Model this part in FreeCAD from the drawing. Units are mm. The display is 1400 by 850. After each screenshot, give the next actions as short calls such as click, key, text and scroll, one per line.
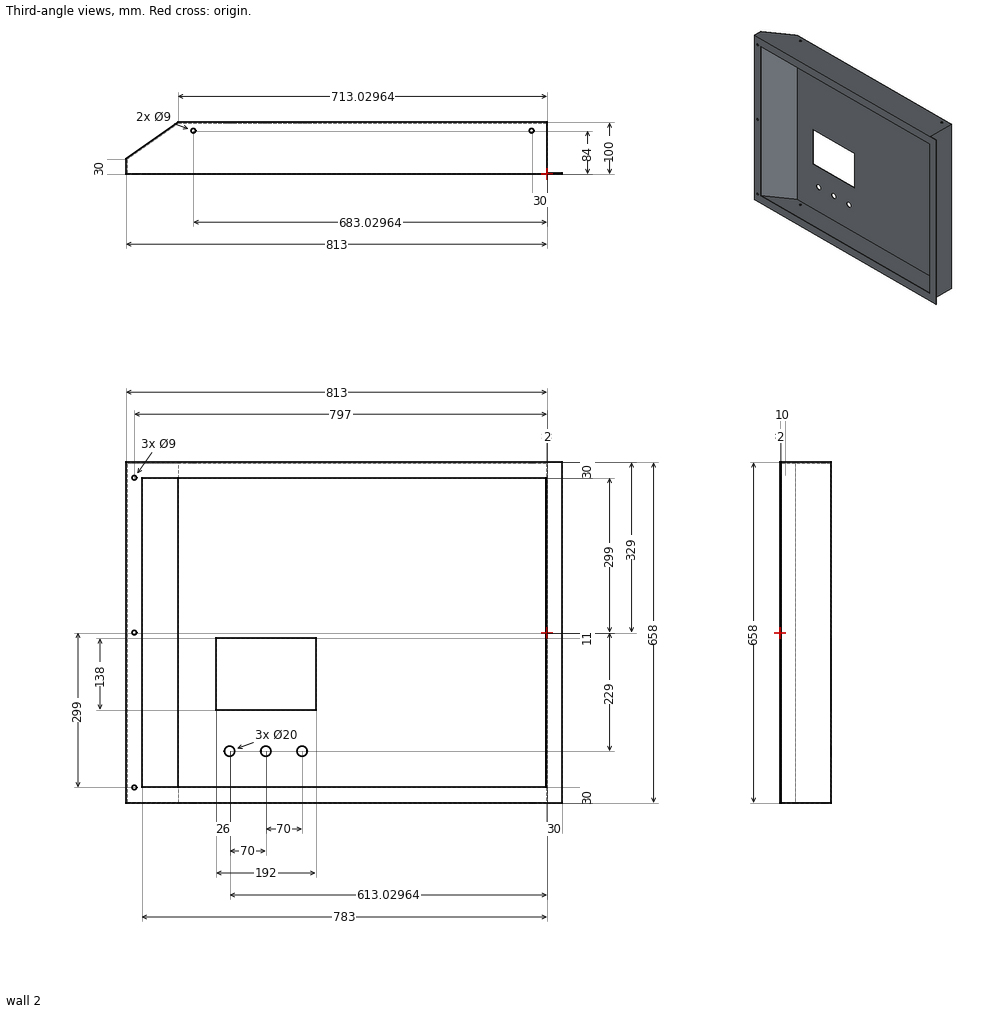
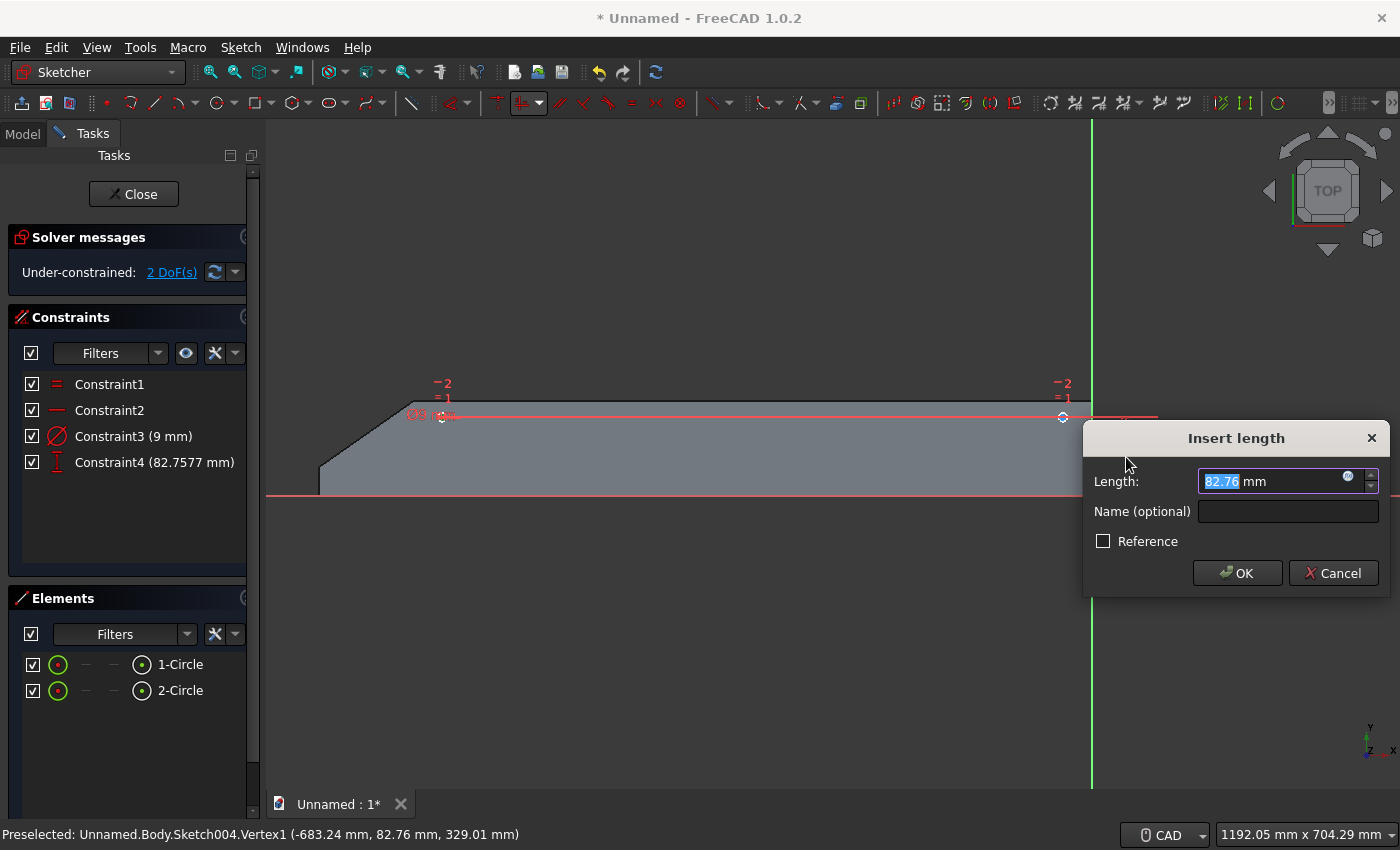
text(84)
key(Return)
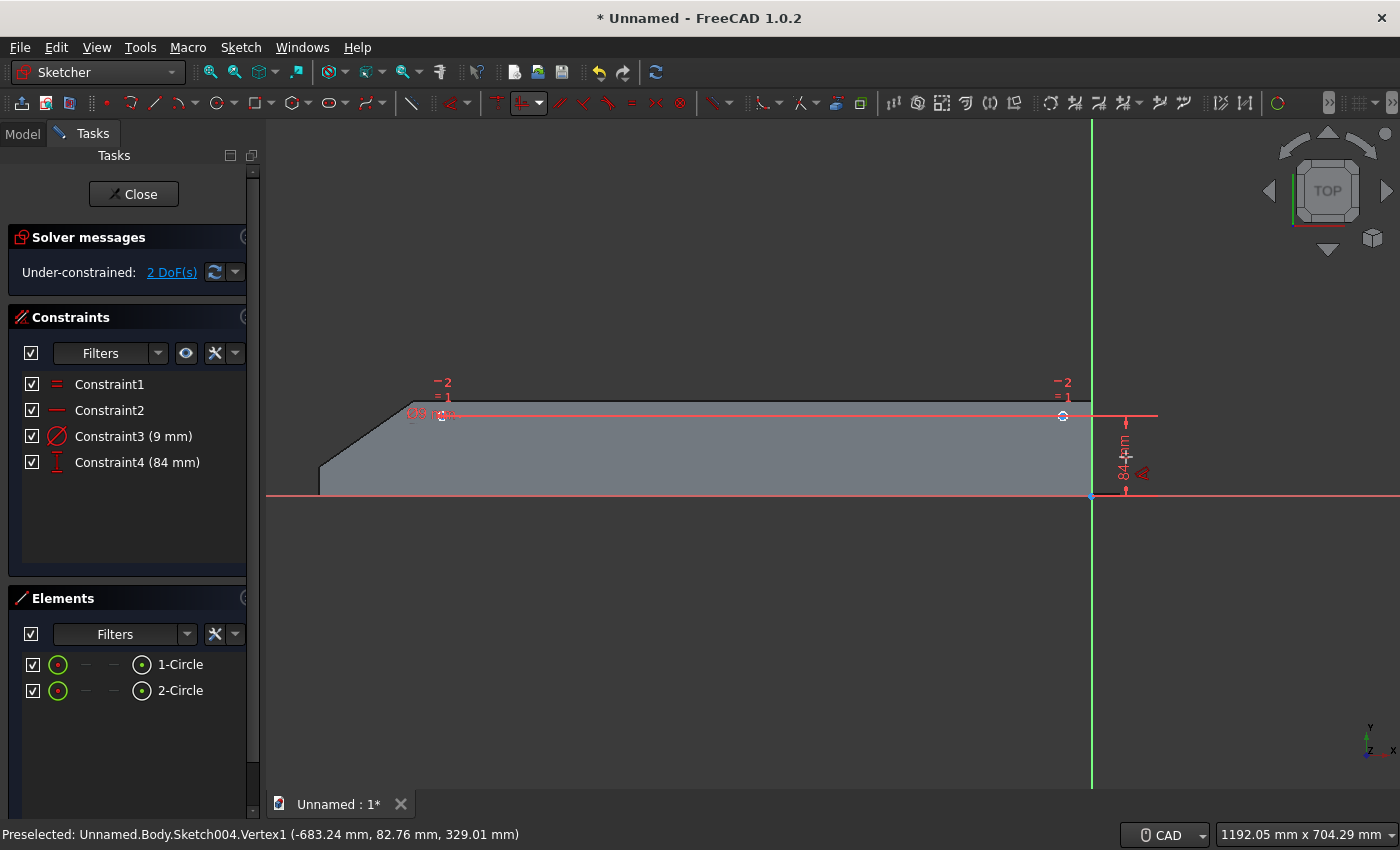
scroll(1063, 416, up, 2)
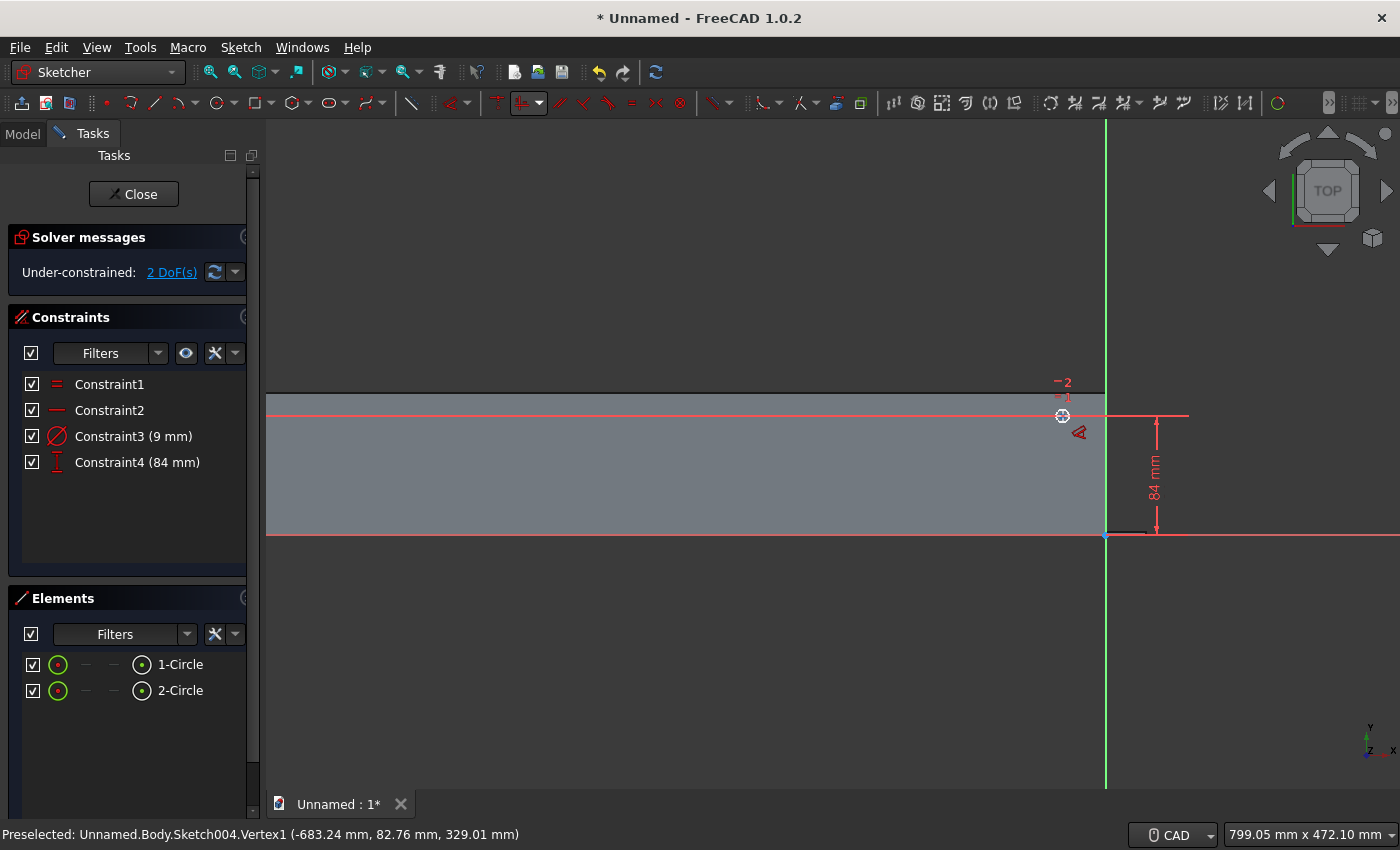
click(1063, 416)
click(1084, 569)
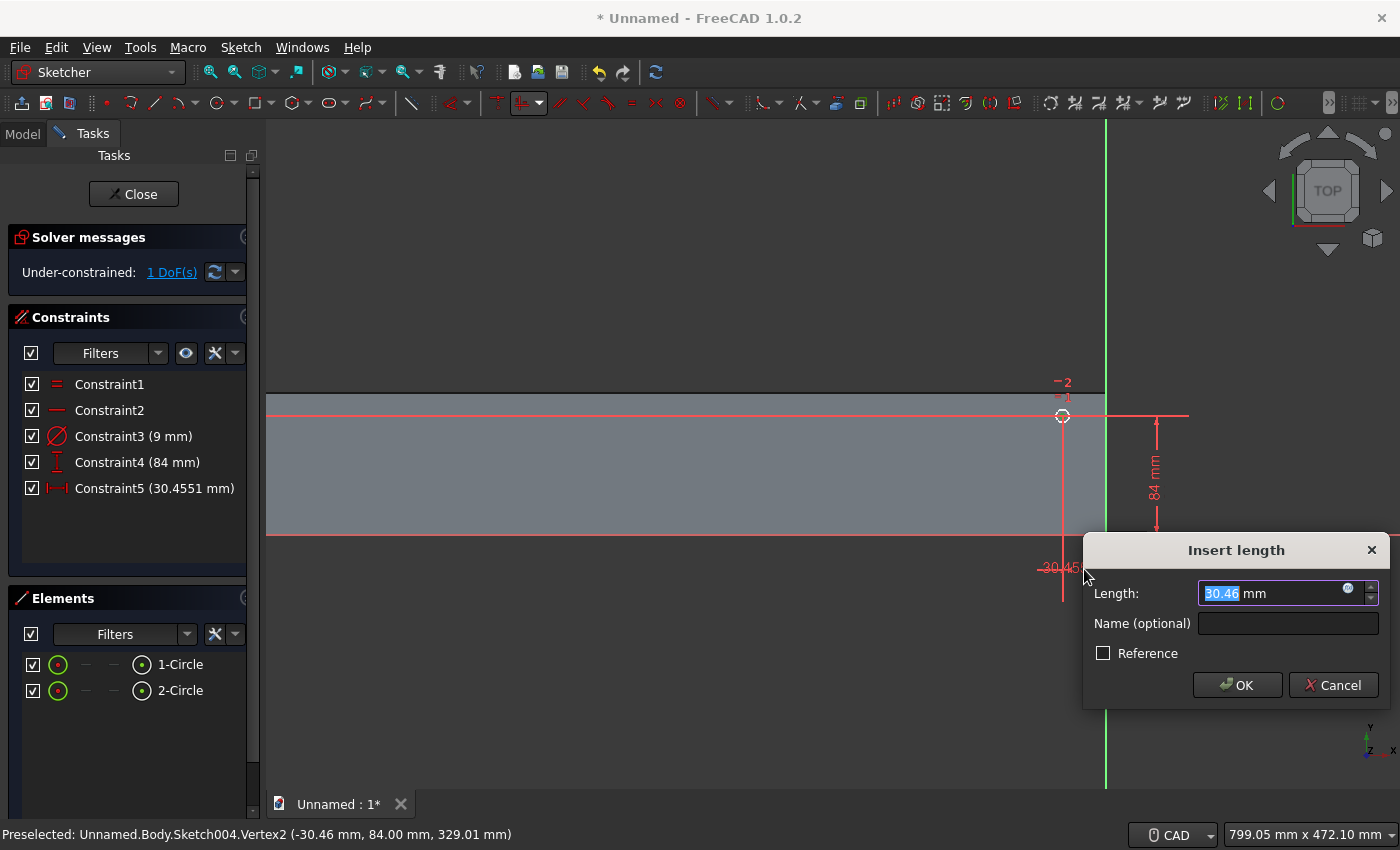
text(30)
key(Return)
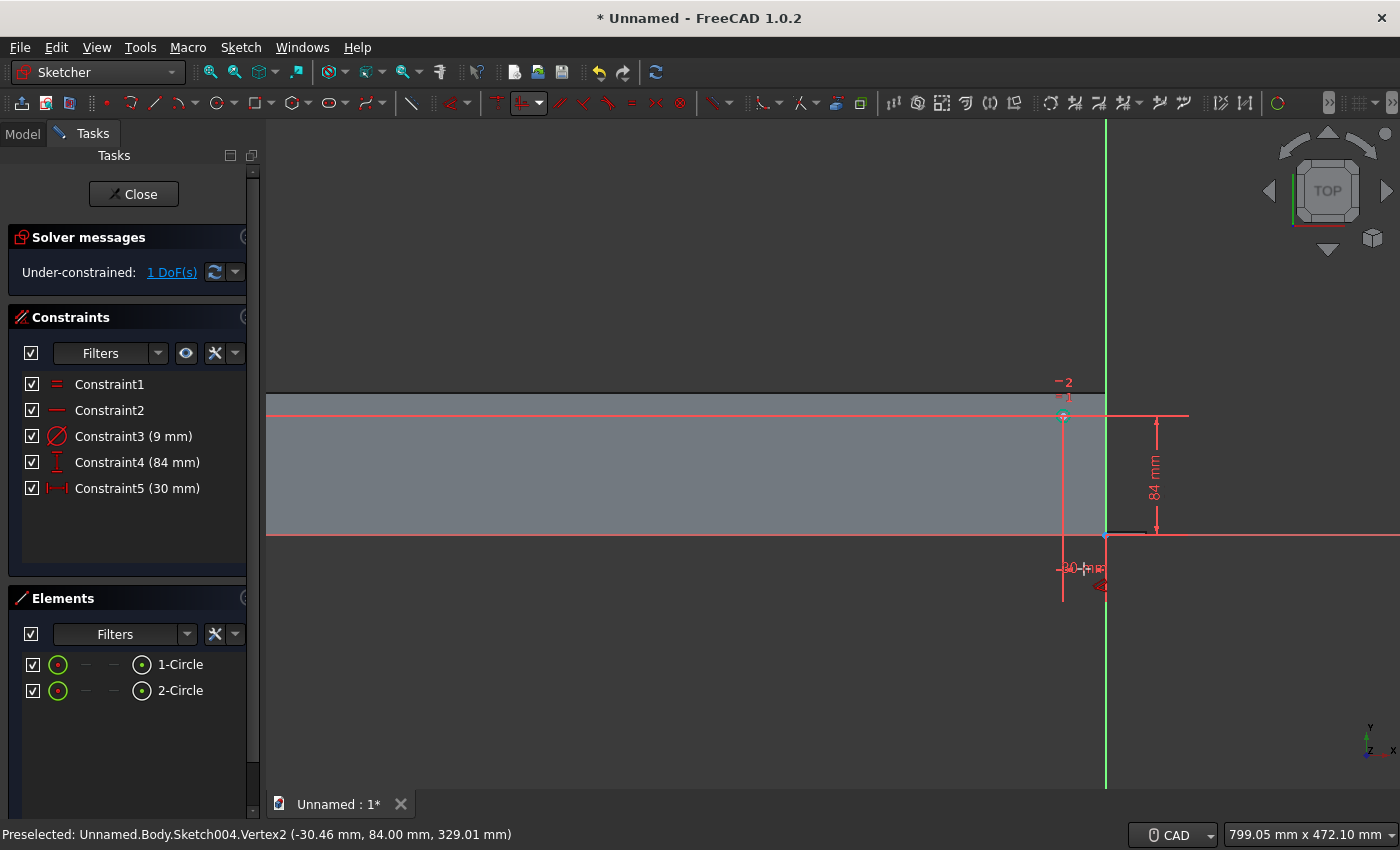
scroll(1062, 416, down, 2)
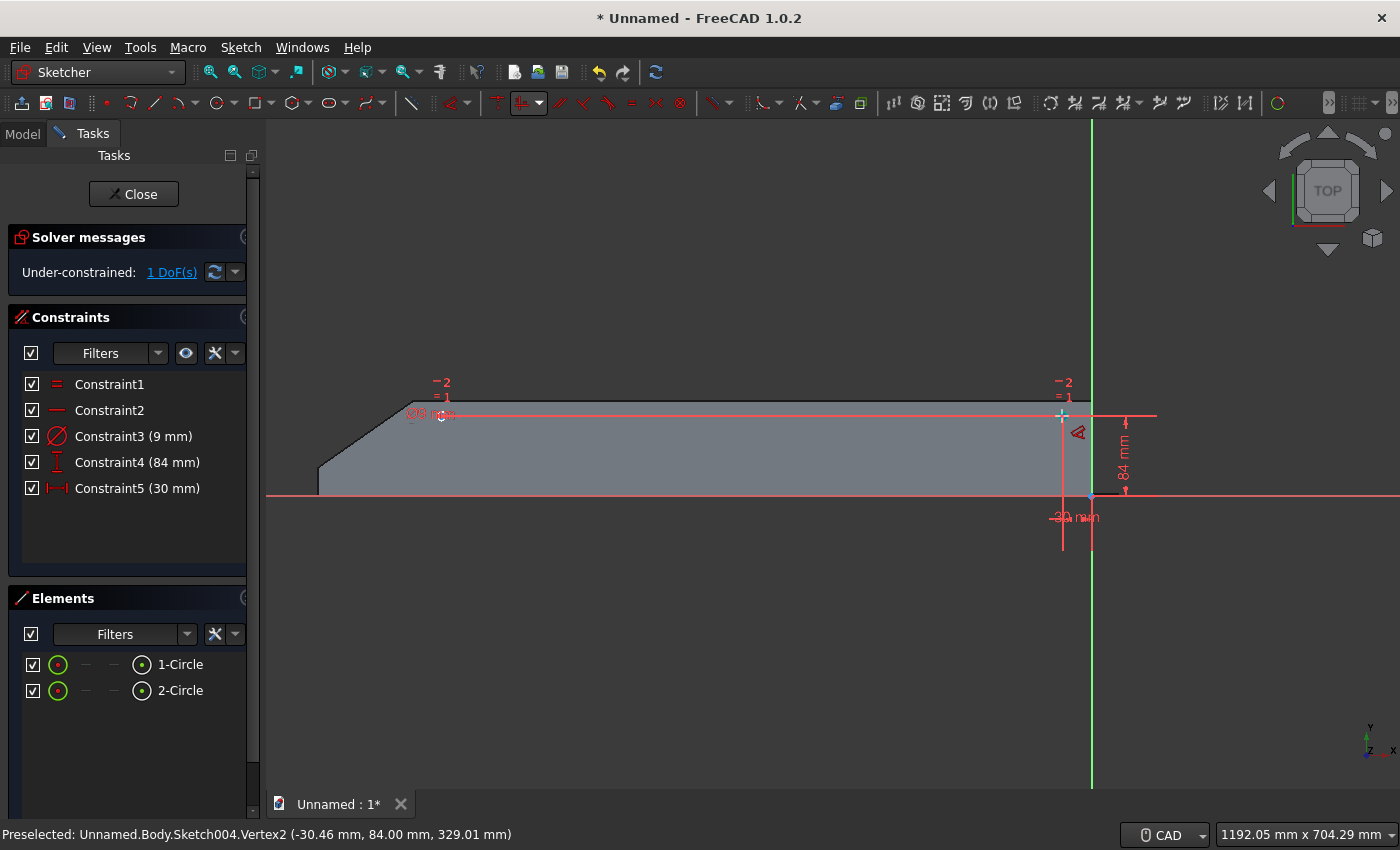
click(442, 416)
click(767, 530)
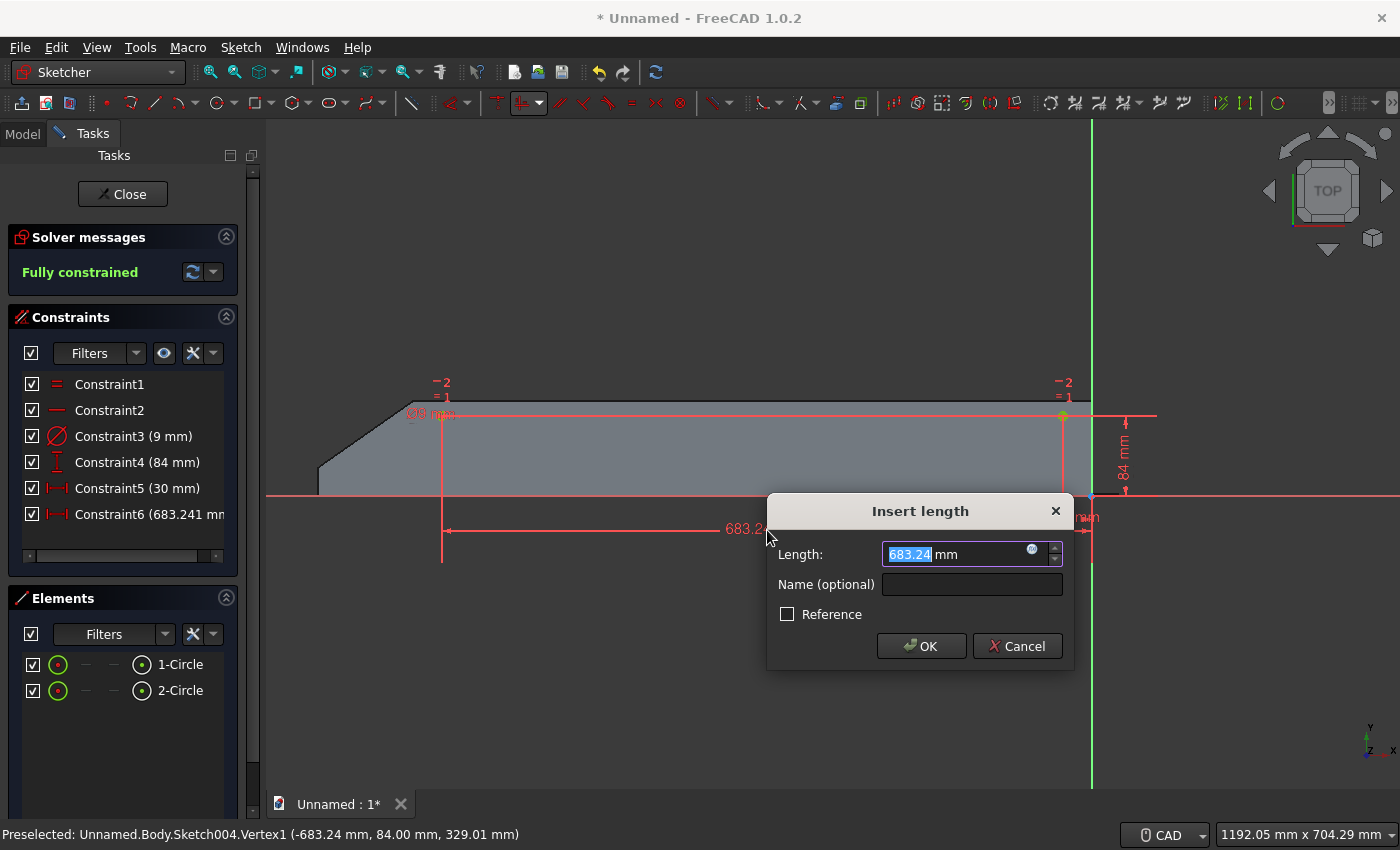
text(683.02964)
key(Return)
key(Escape)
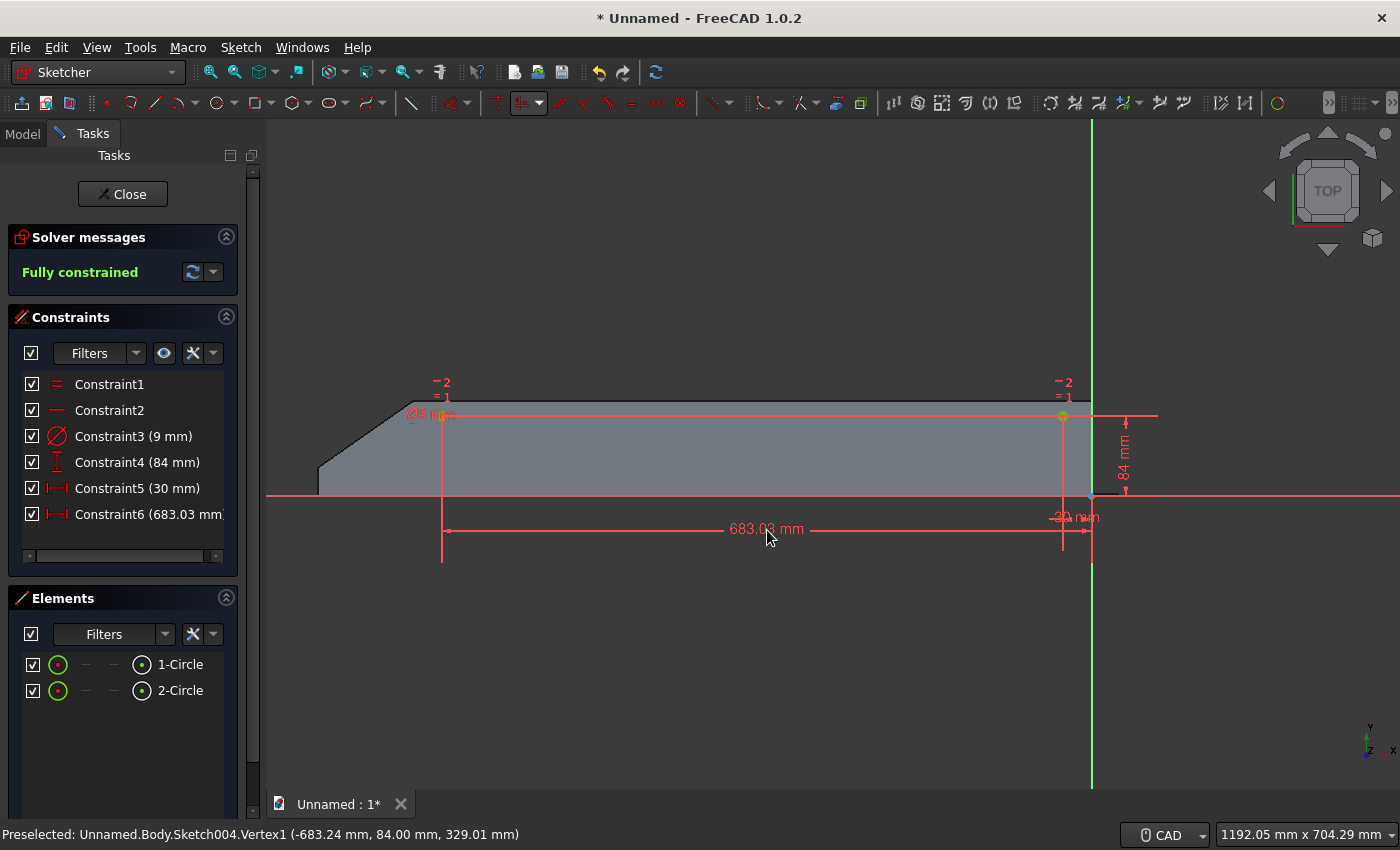
click(123, 194)